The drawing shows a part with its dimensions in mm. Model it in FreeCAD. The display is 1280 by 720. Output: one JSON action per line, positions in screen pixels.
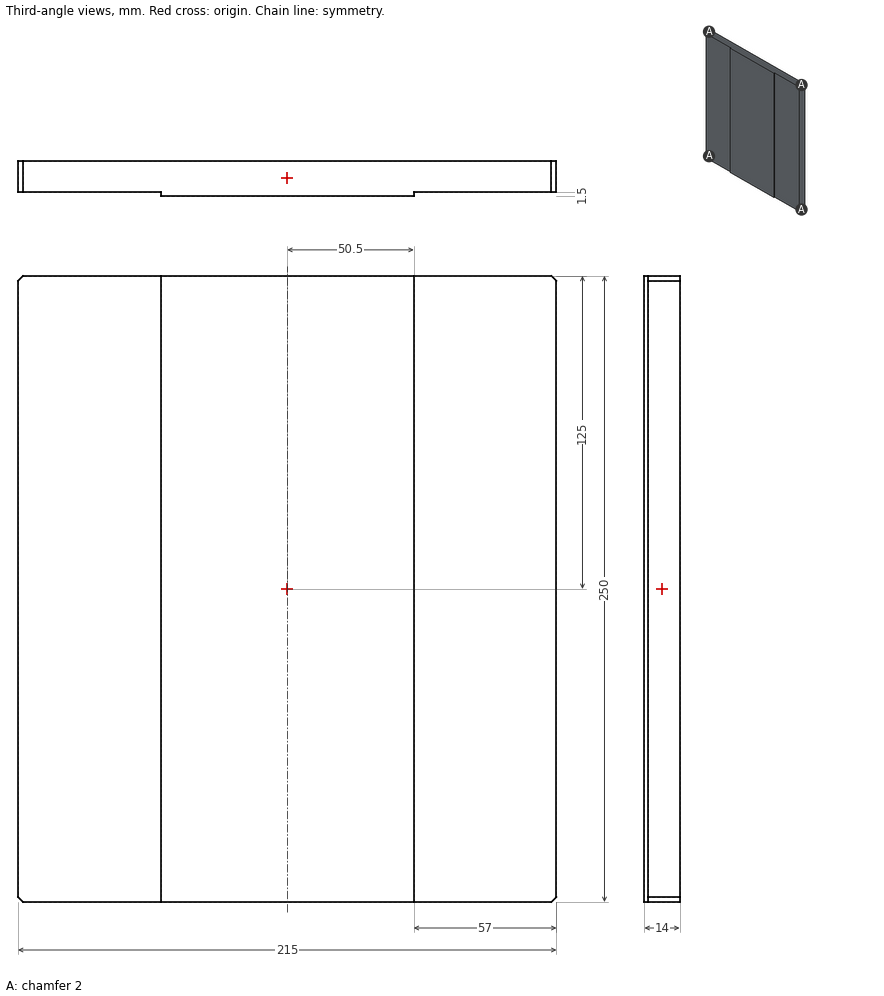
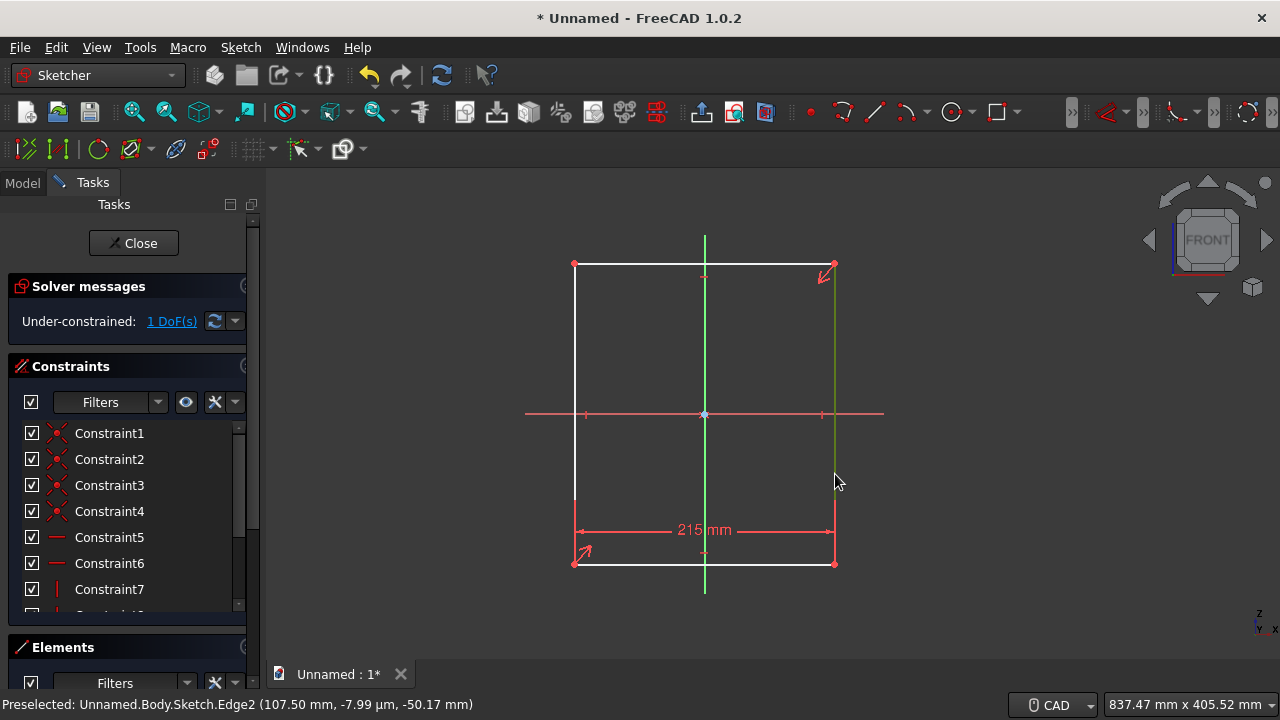
{"action": "key", "text": "i"}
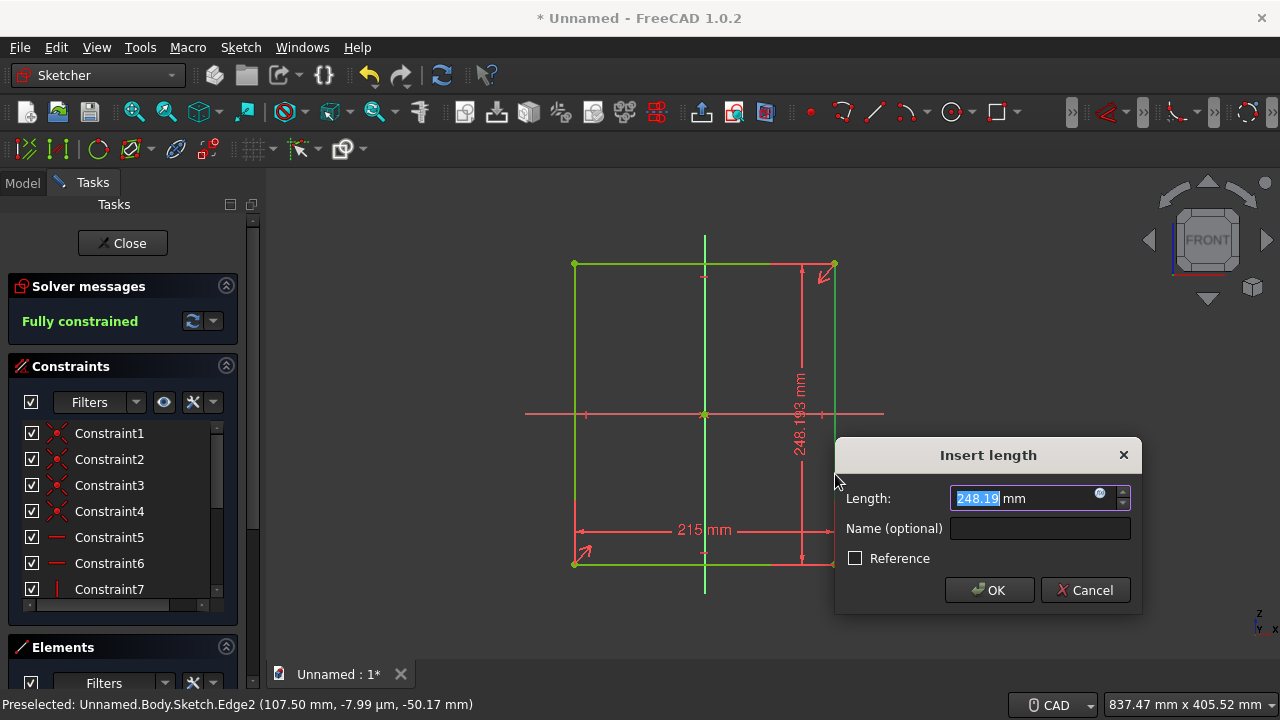
{"action": "type", "text": "250"}
{"action": "key", "text": "Return"}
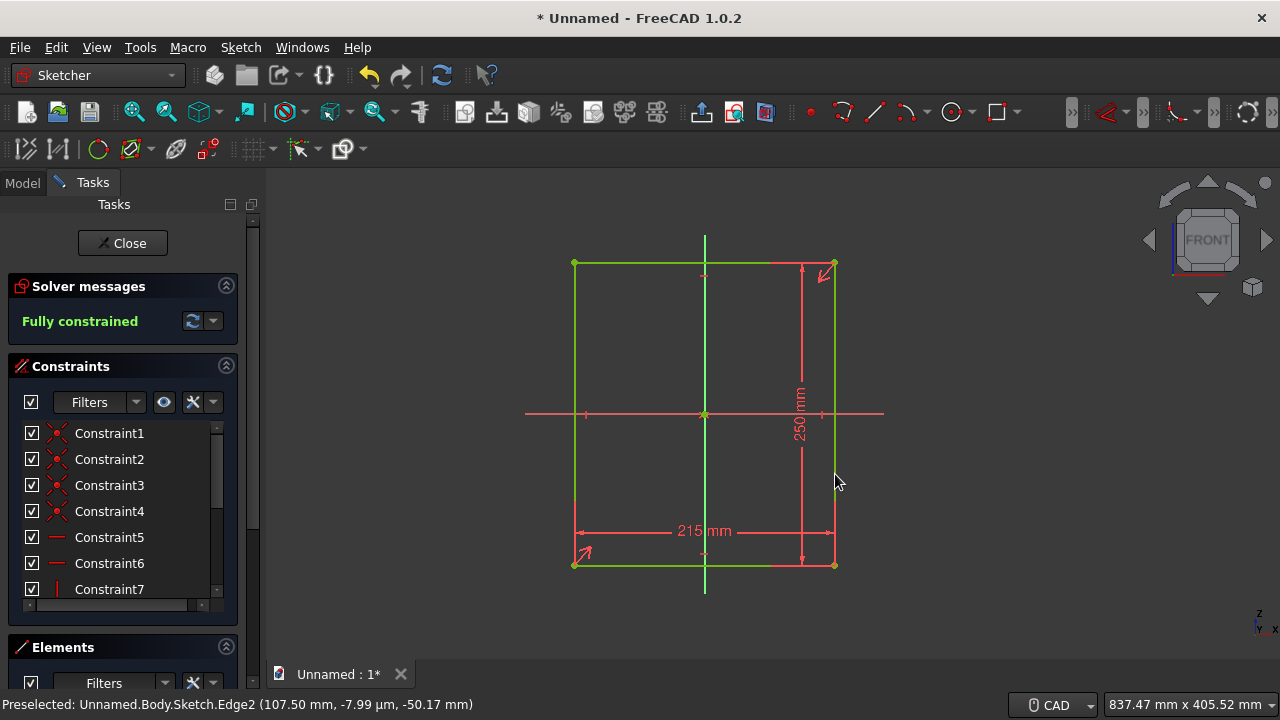
{"action": "left_click", "coordinate": [123, 243]}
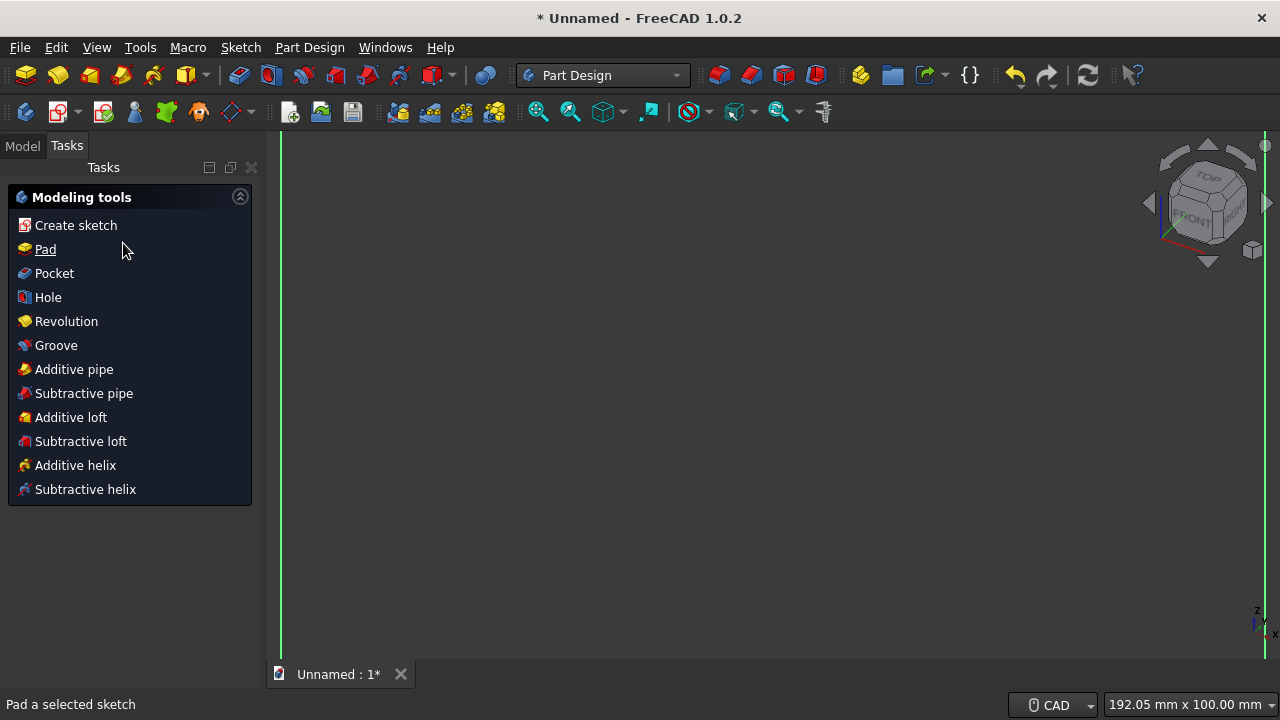
{"action": "left_click", "coordinate": [26, 76]}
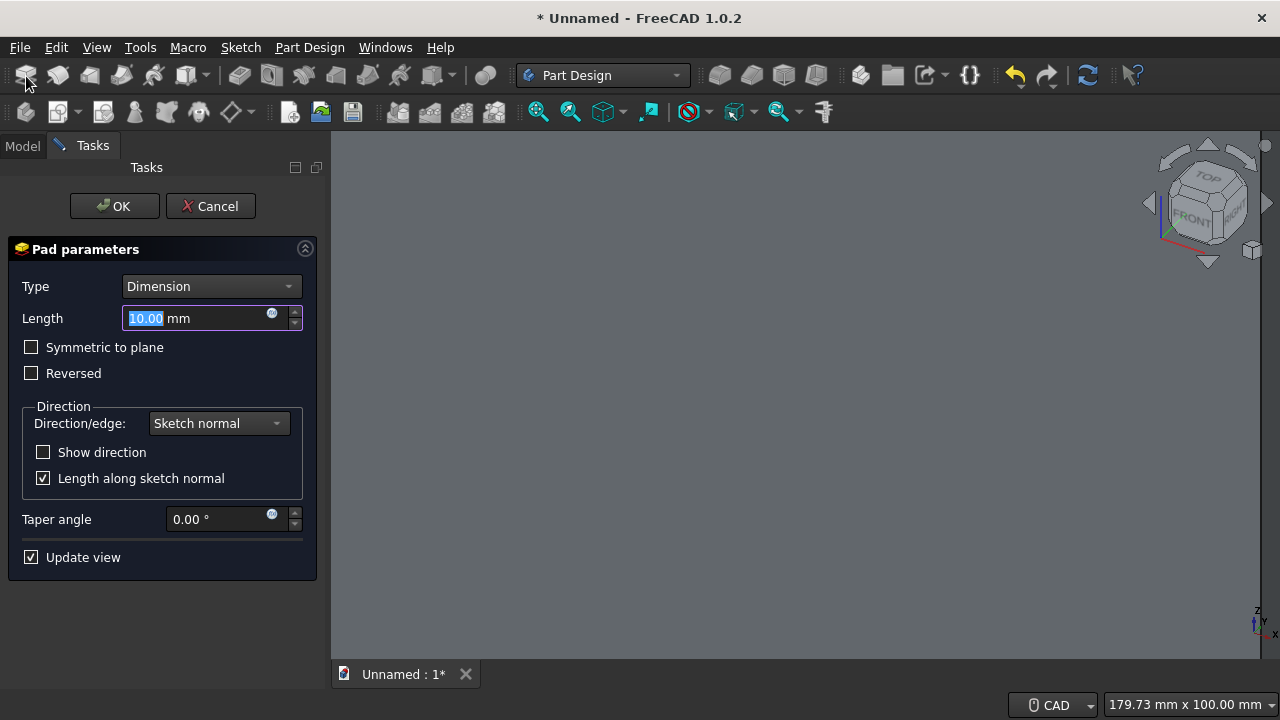
{"action": "type", "text": "14"}
{"action": "key", "text": "Tab"}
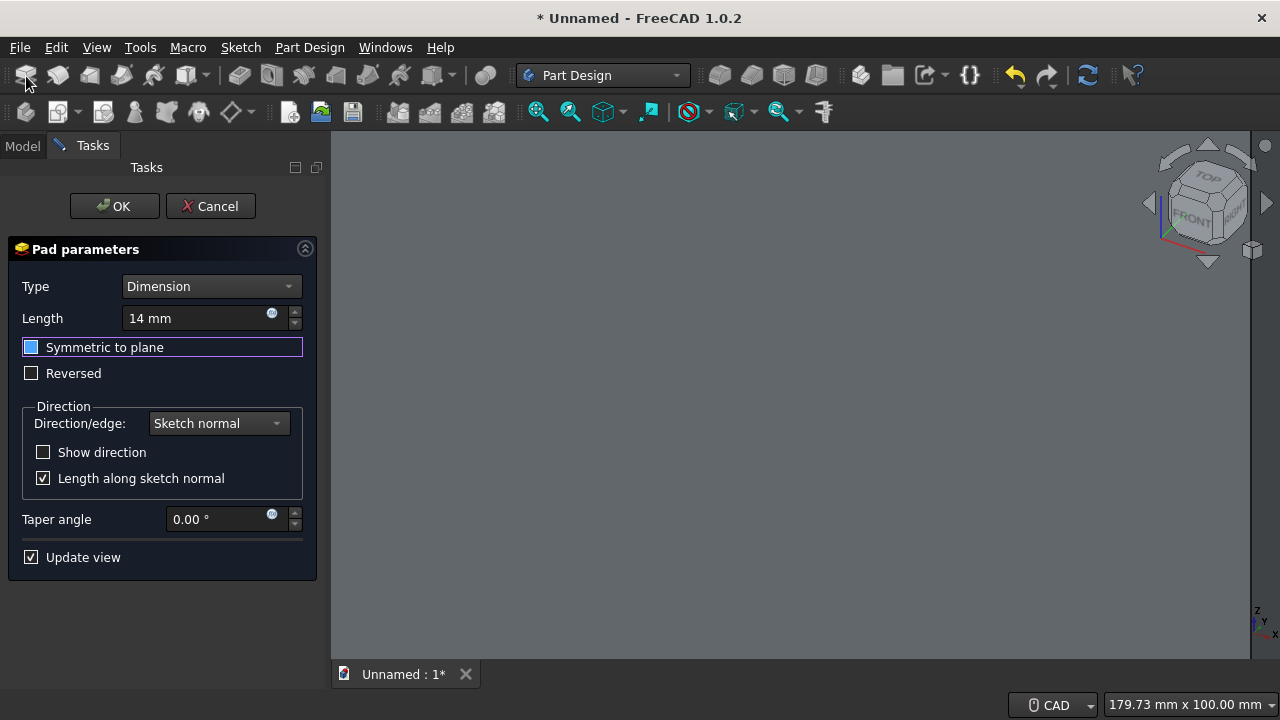
{"action": "left_click", "coordinate": [30, 347]}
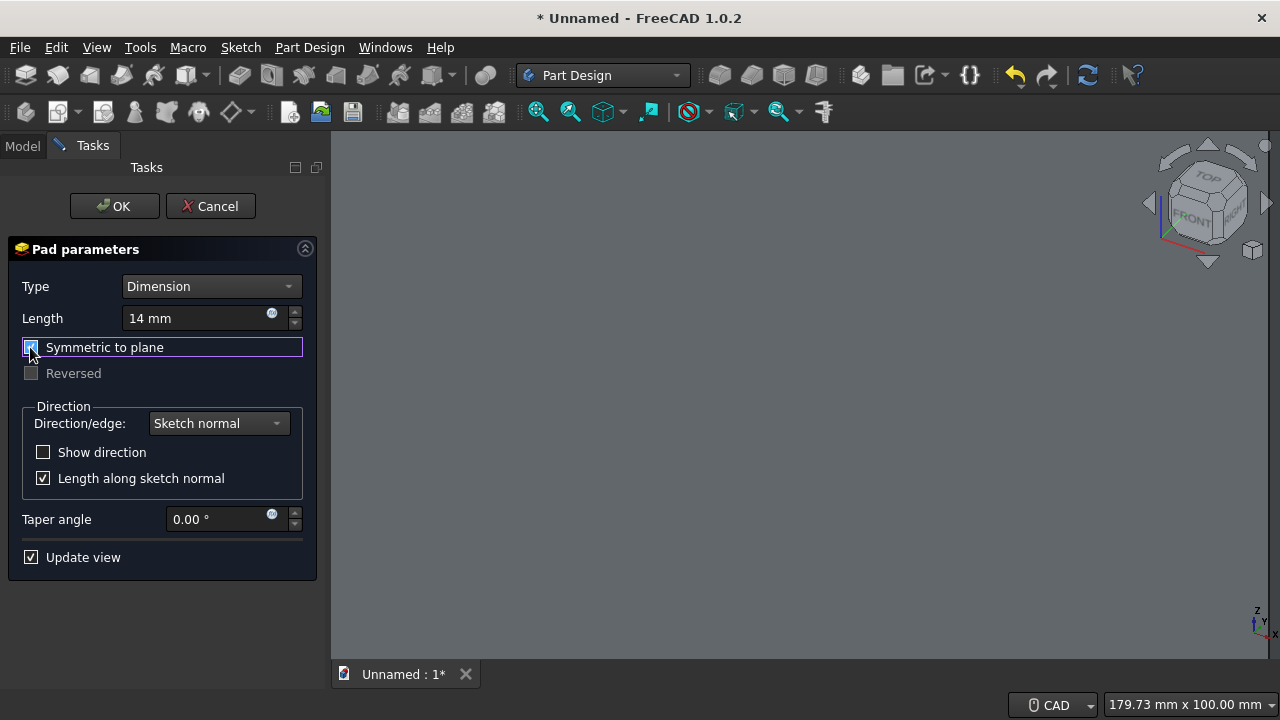
{"action": "left_click", "coordinate": [115, 206]}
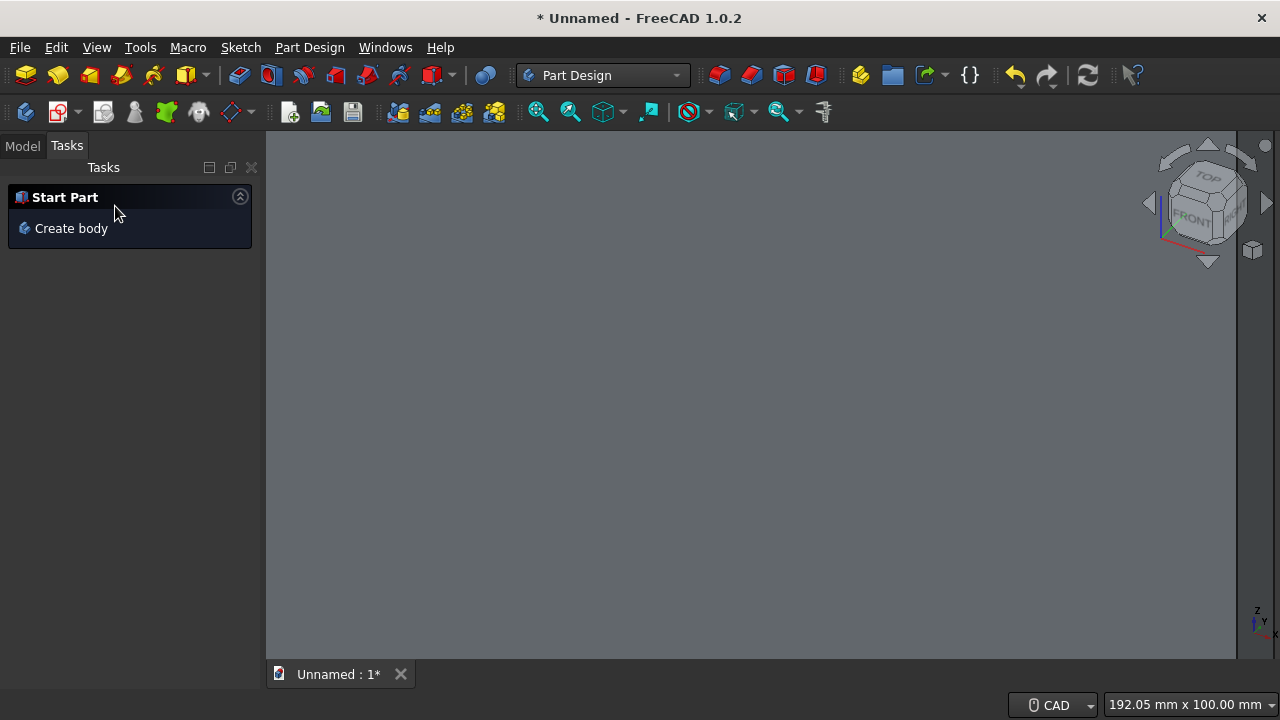
{"action": "key", "text": "v f"}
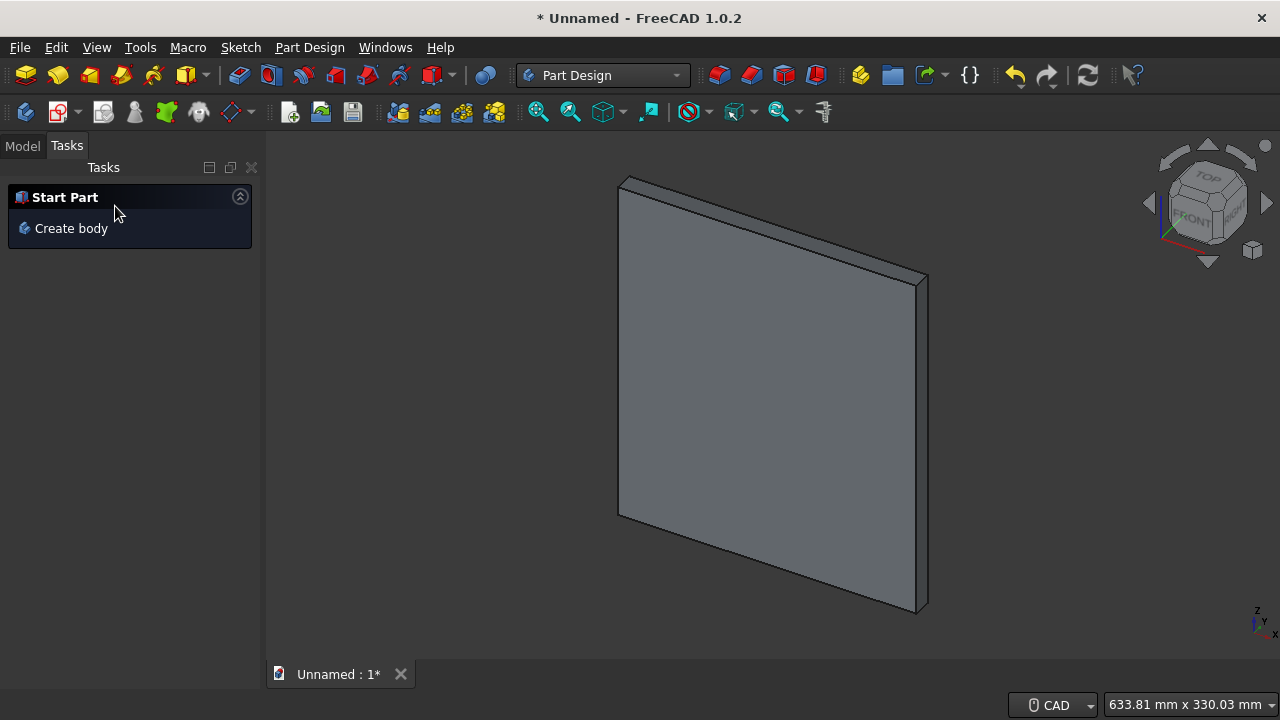
{"action": "left_click", "coordinate": [767, 400]}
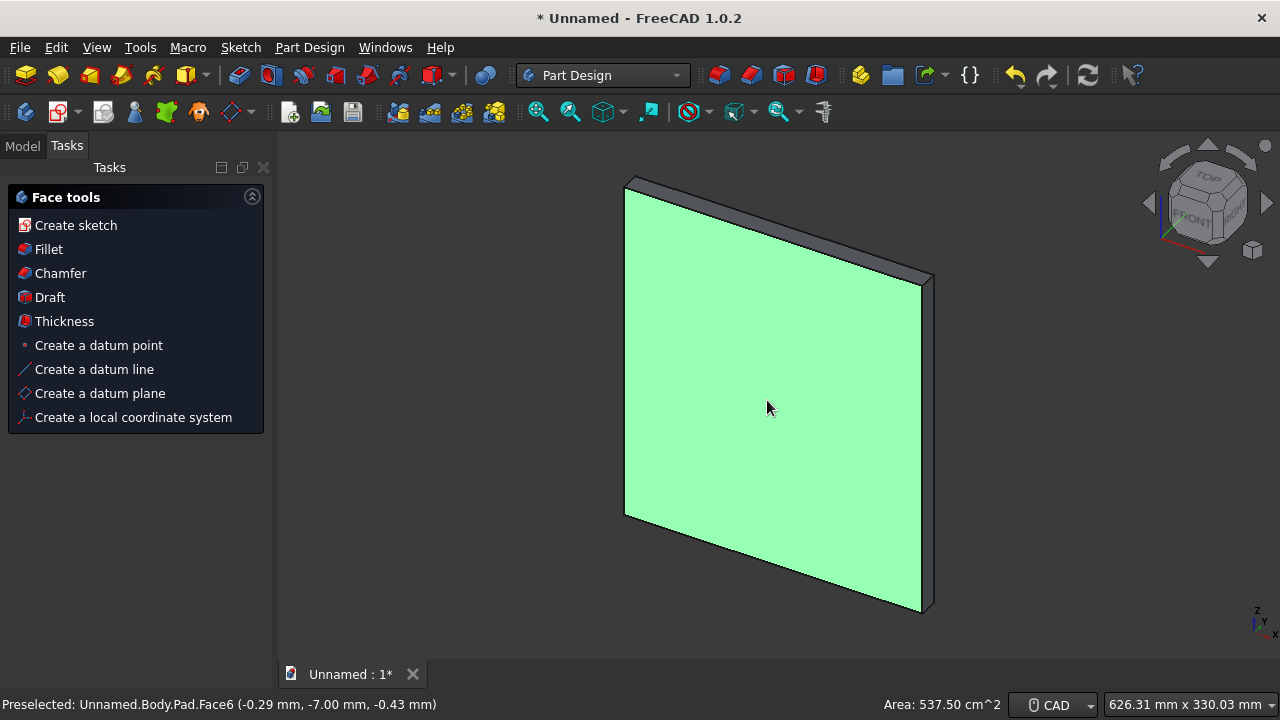
{"action": "left_click", "coordinate": [58, 112]}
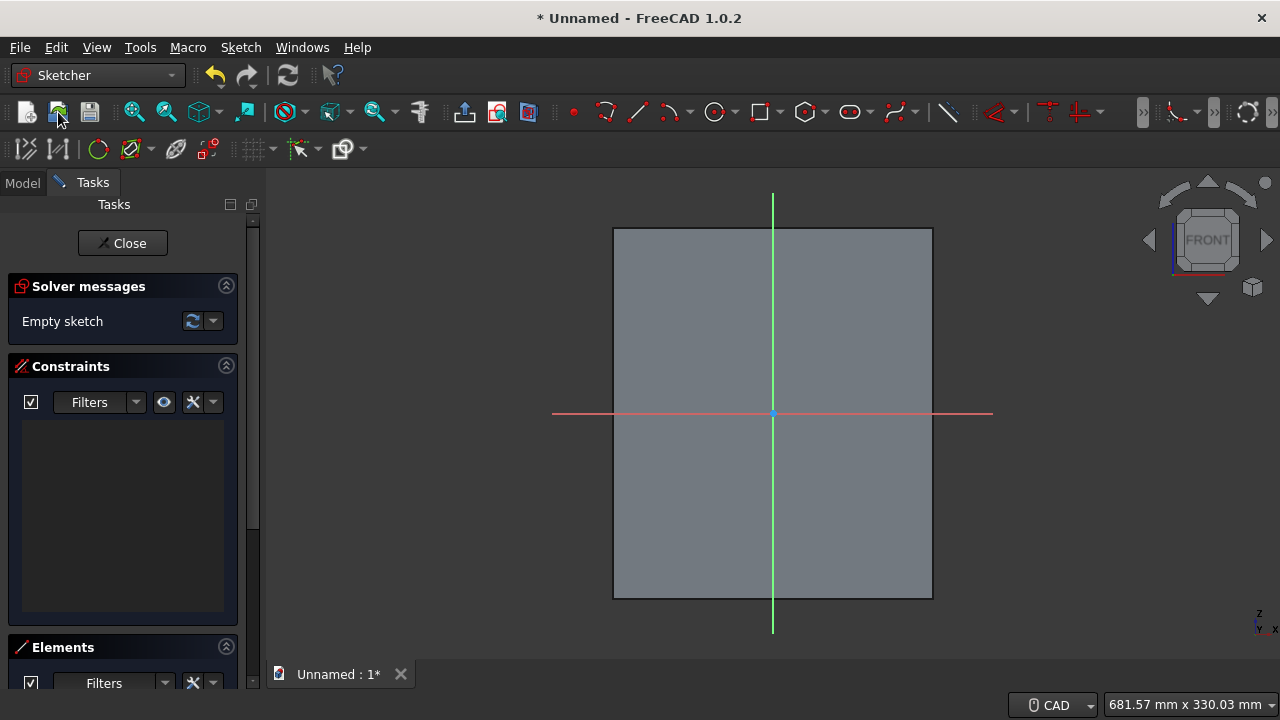
{"action": "key", "text": "g r"}